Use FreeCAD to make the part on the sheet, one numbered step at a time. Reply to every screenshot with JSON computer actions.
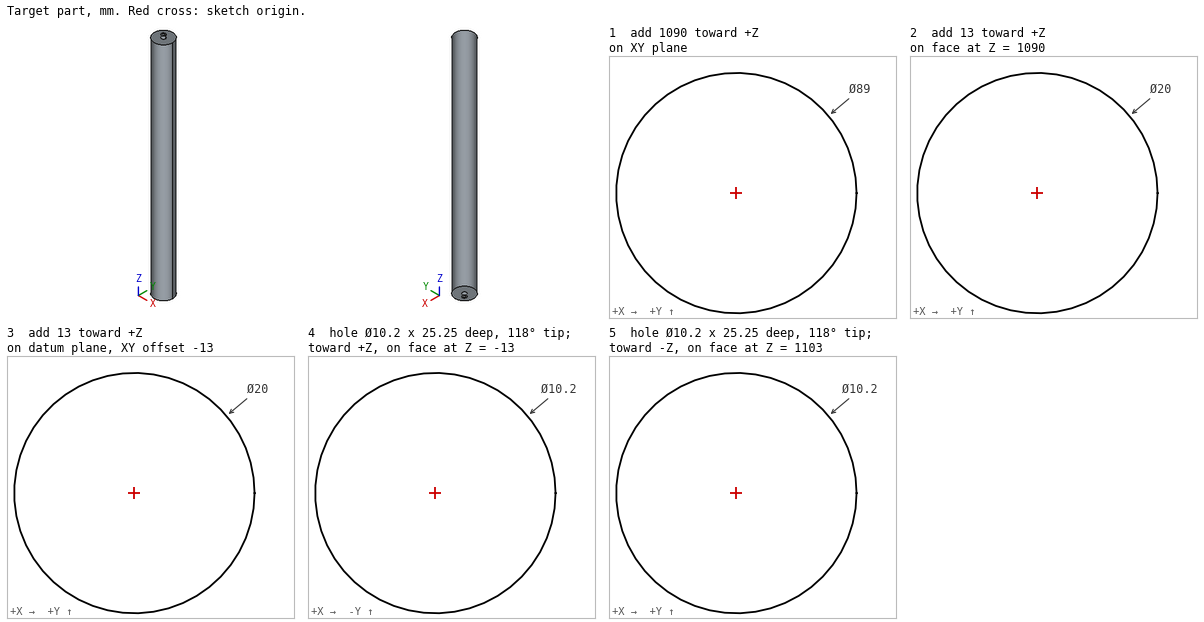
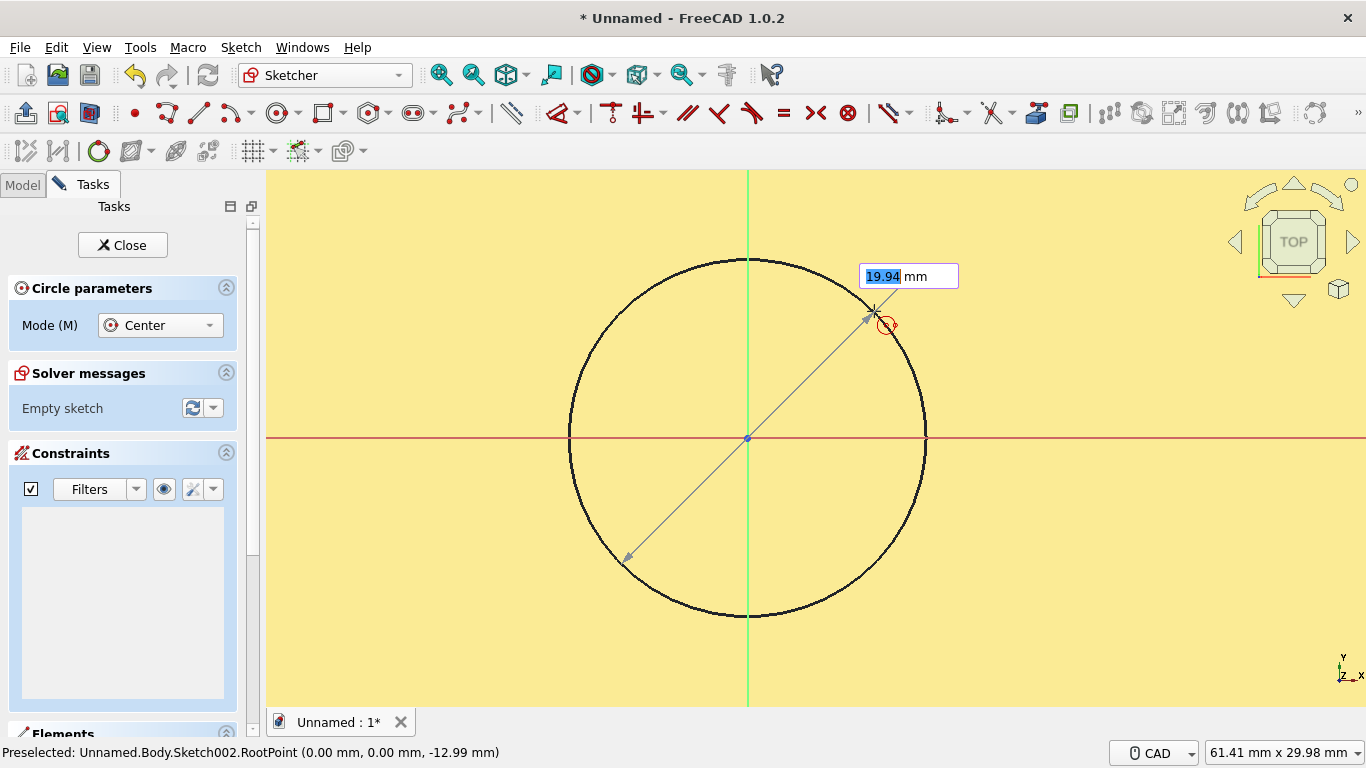
{"action": "type", "text": "20"}
{"action": "key", "text": "Return"}
{"action": "key", "text": "Escape"}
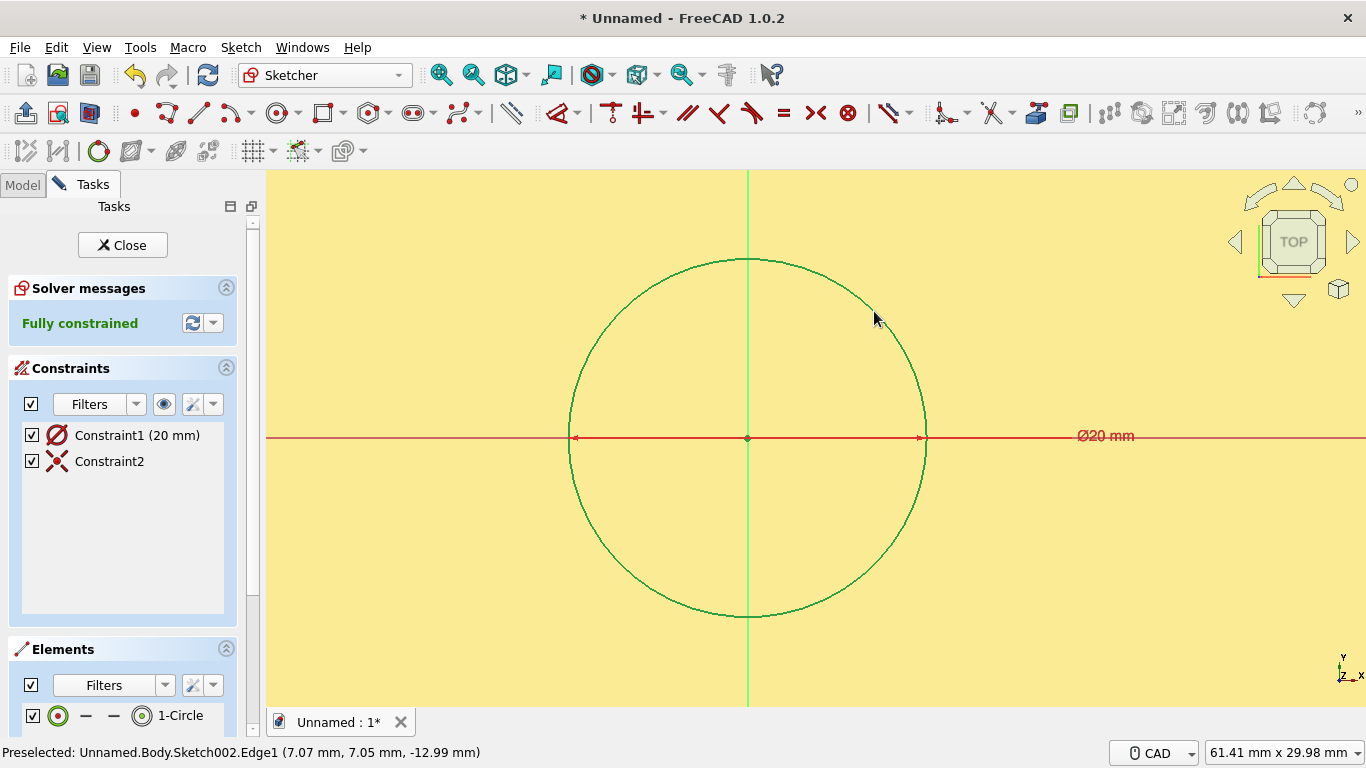
{"action": "left_click", "coordinate": [123, 245]}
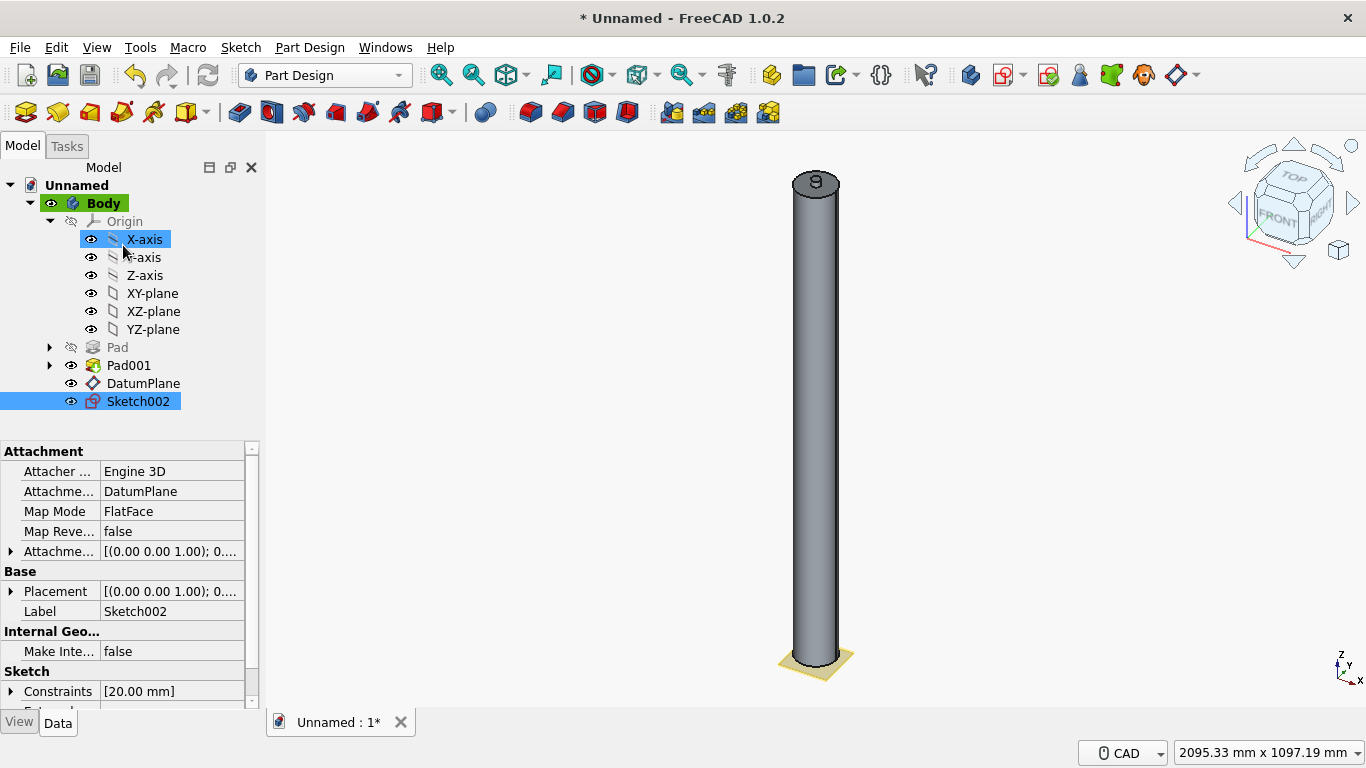
{"action": "left_click", "coordinate": [26, 112]}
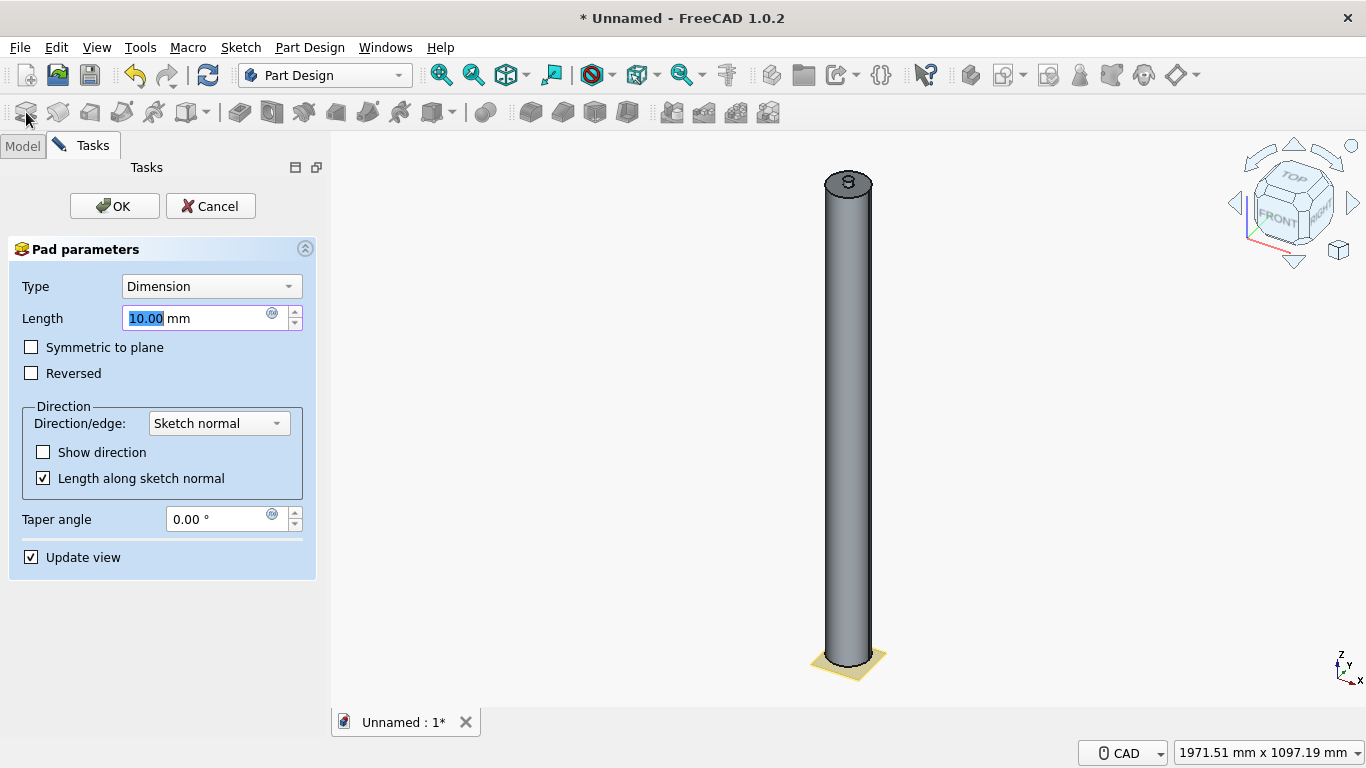
{"action": "type", "text": "13"}
{"action": "key", "text": "Tab"}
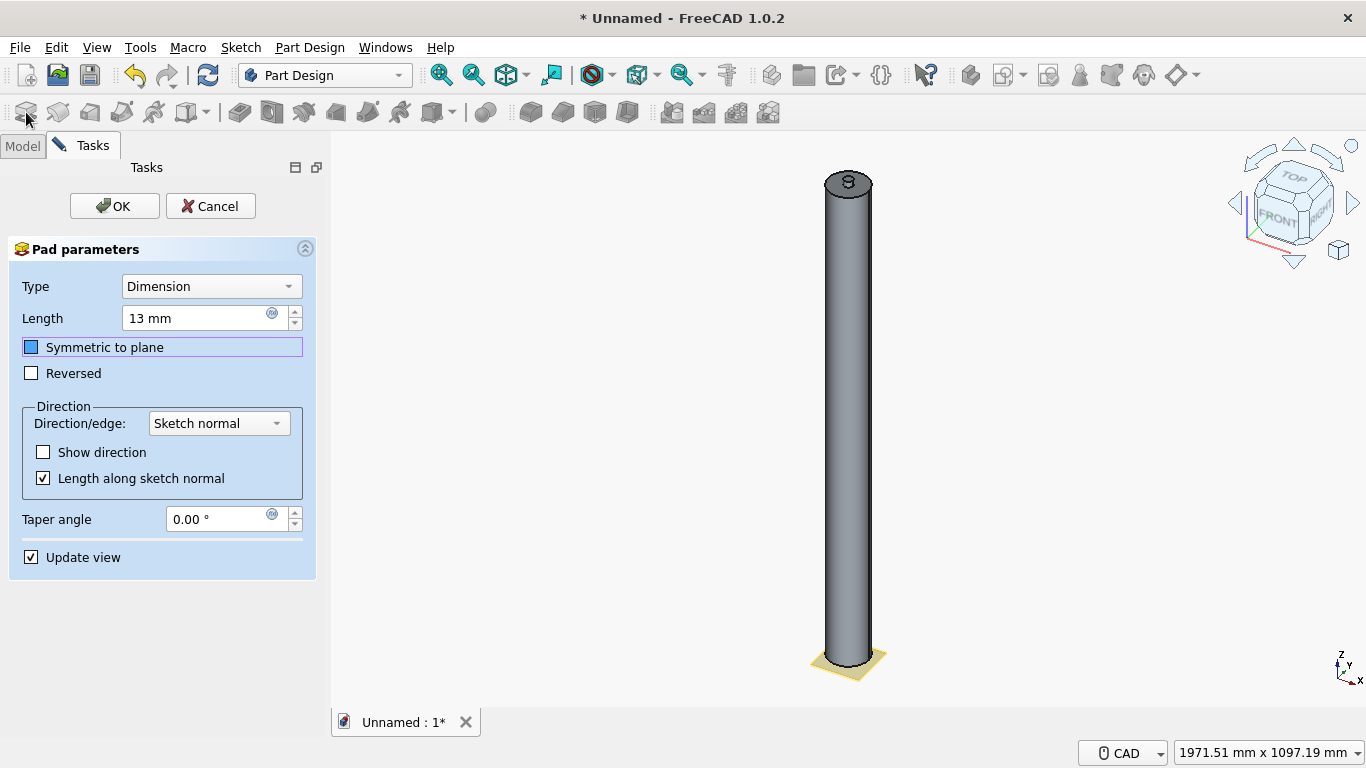
{"action": "left_click", "coordinate": [115, 206]}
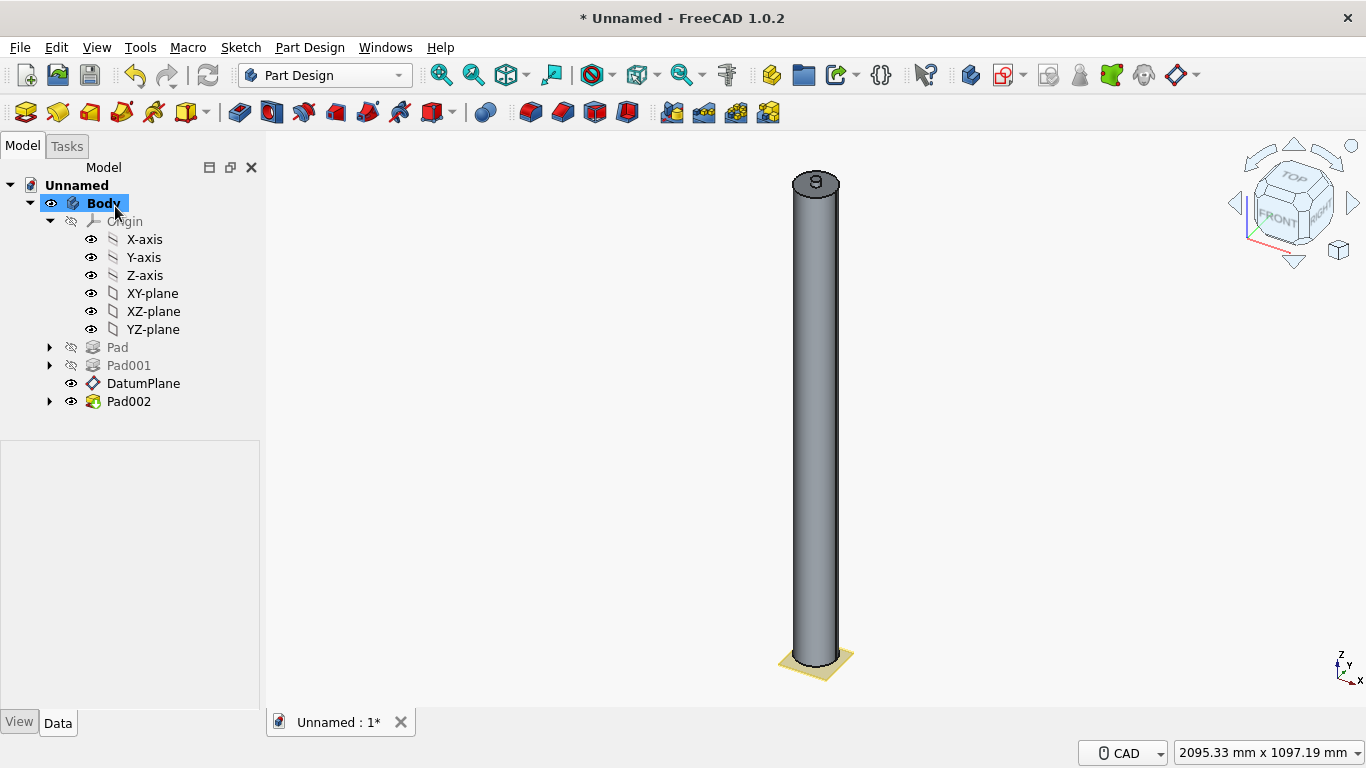
{"action": "left_click", "coordinate": [116, 383]}
{"action": "key", "text": "space"}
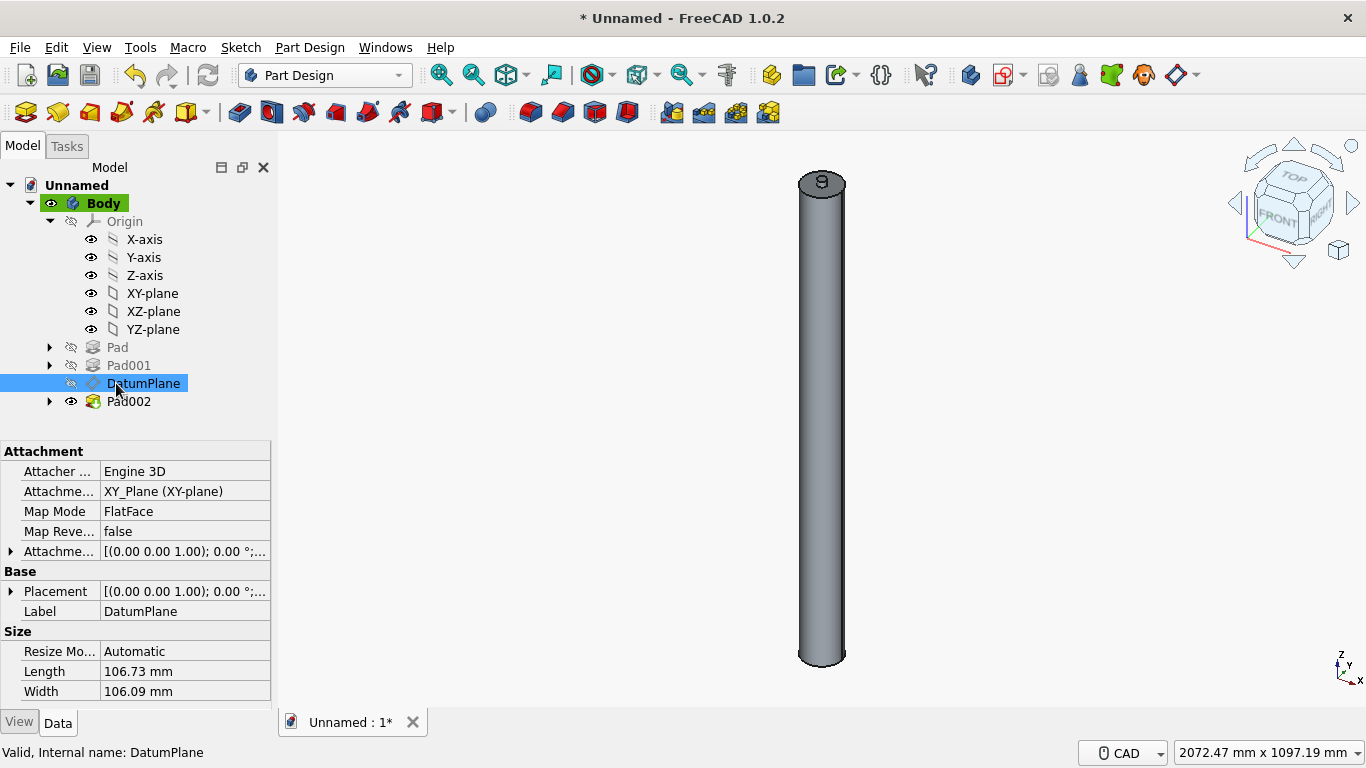
{"action": "key", "text": "5"}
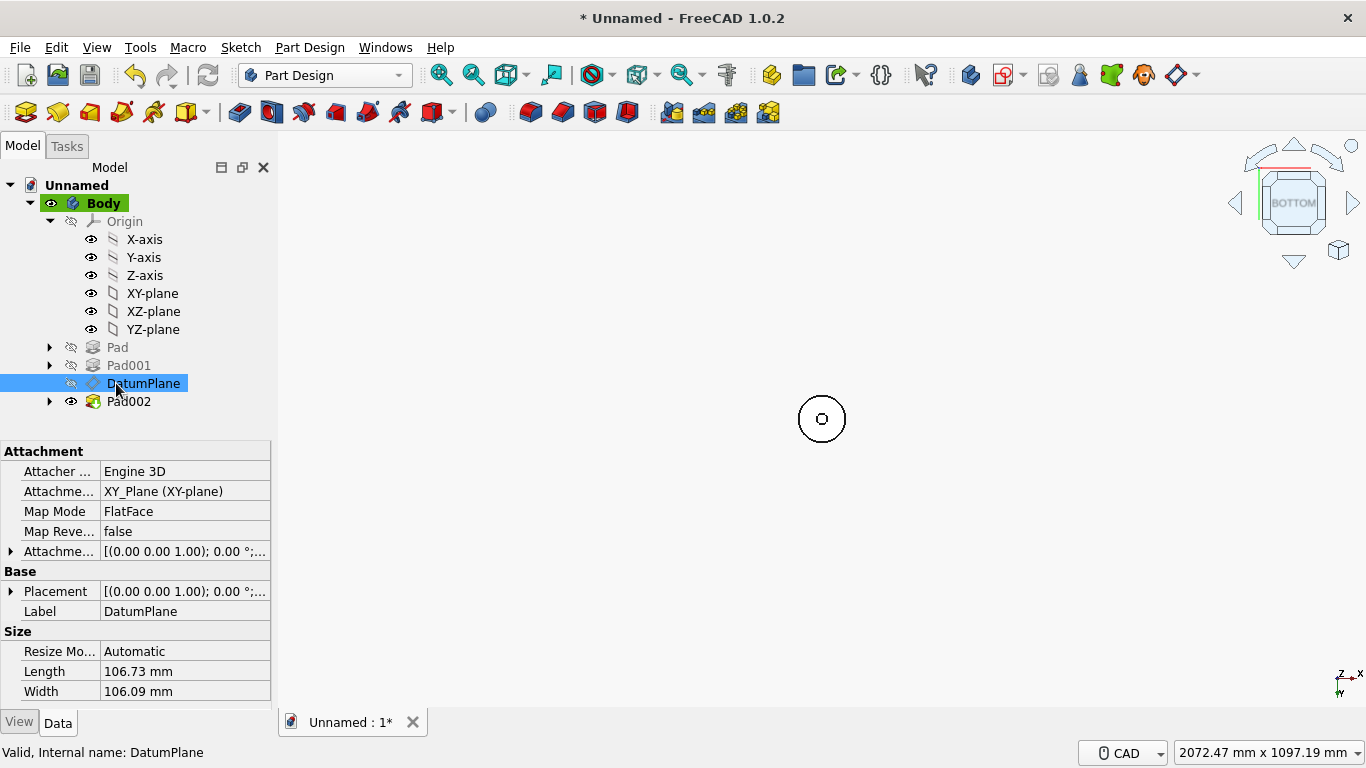
{"action": "left_click", "coordinate": [442, 76]}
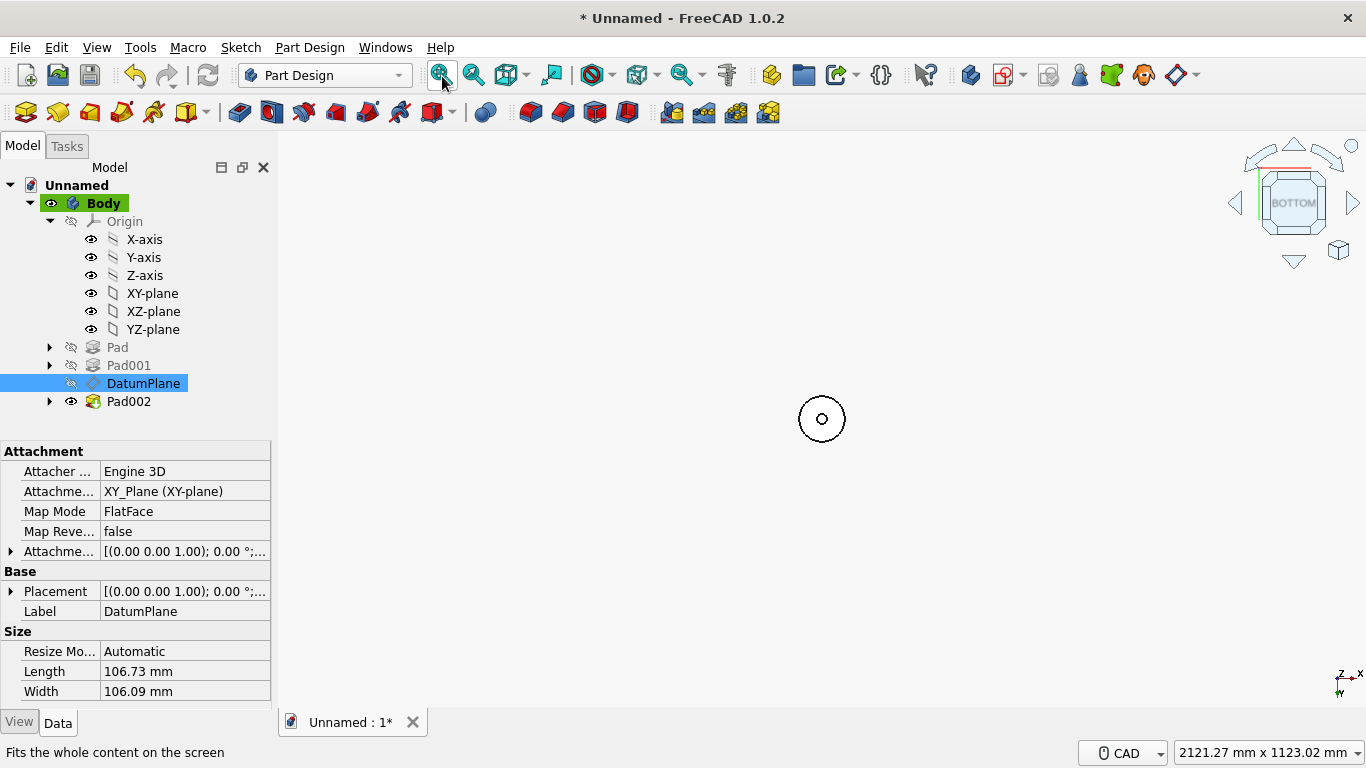
{"action": "scroll", "coordinate": [822, 418], "scroll_direction": "up", "scroll_amount": 5}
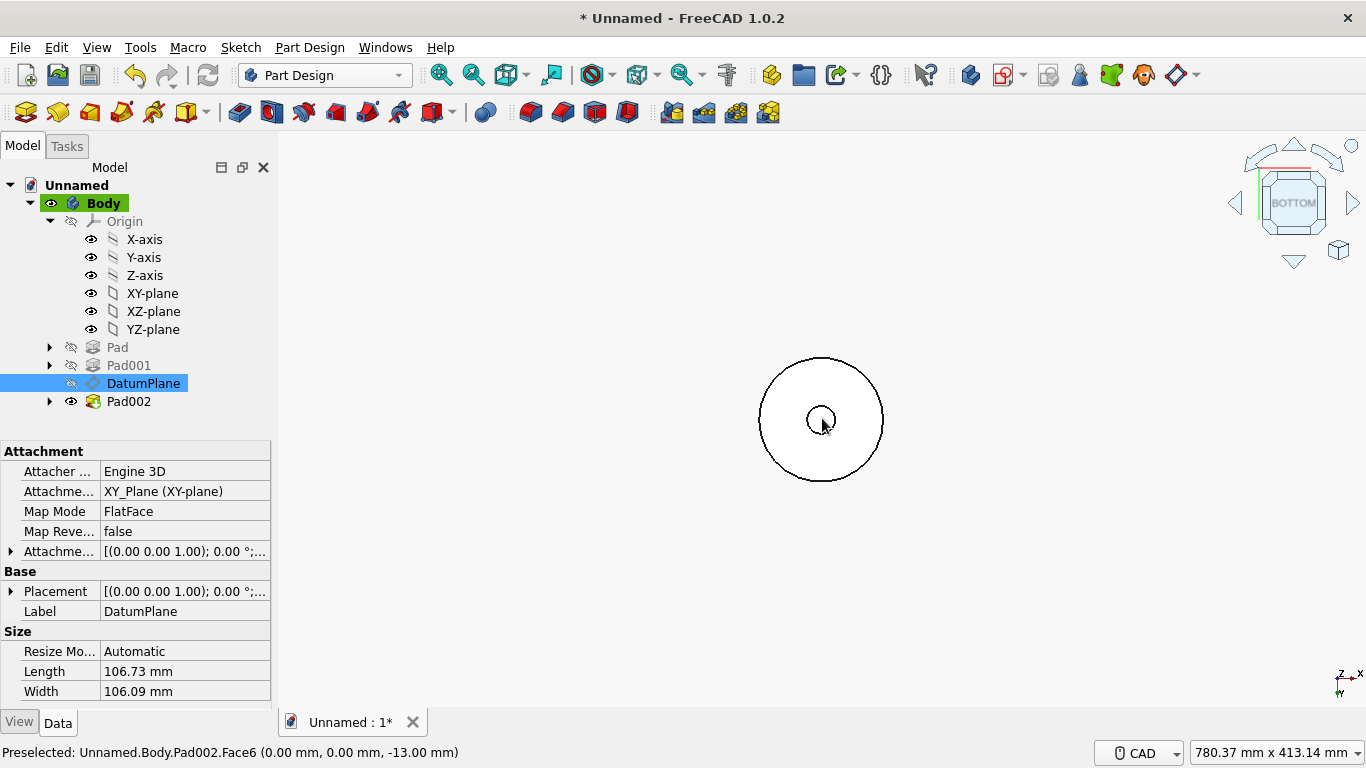
{"action": "left_click", "coordinate": [821, 419]}